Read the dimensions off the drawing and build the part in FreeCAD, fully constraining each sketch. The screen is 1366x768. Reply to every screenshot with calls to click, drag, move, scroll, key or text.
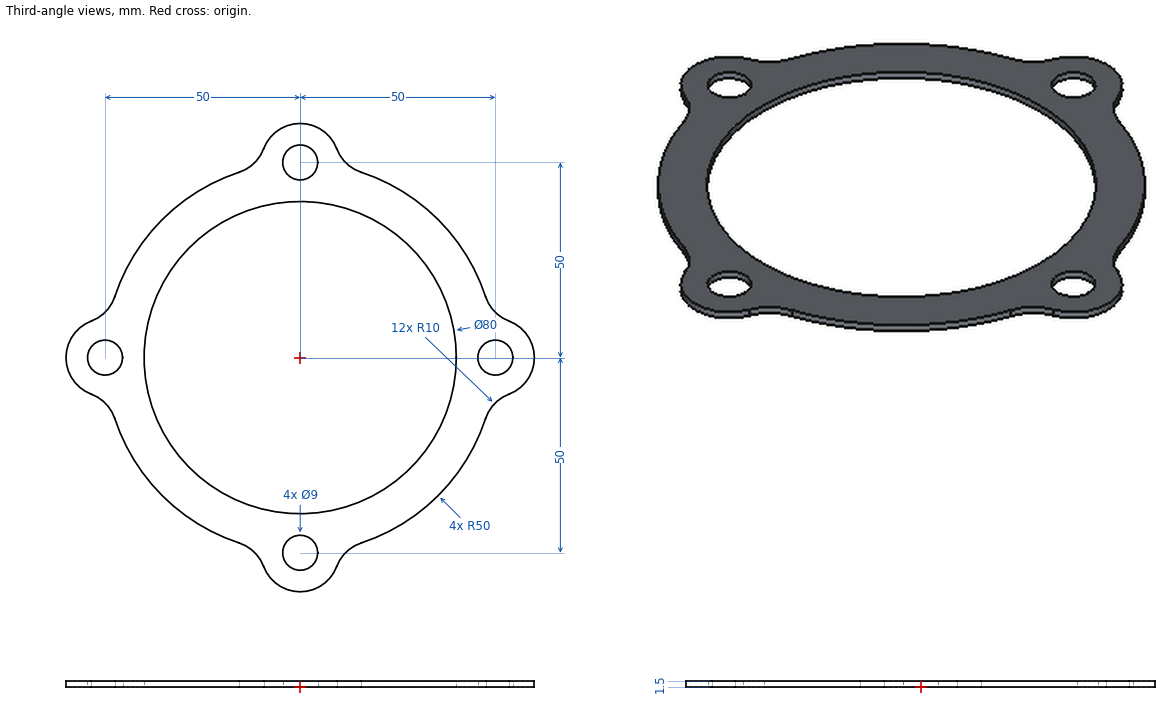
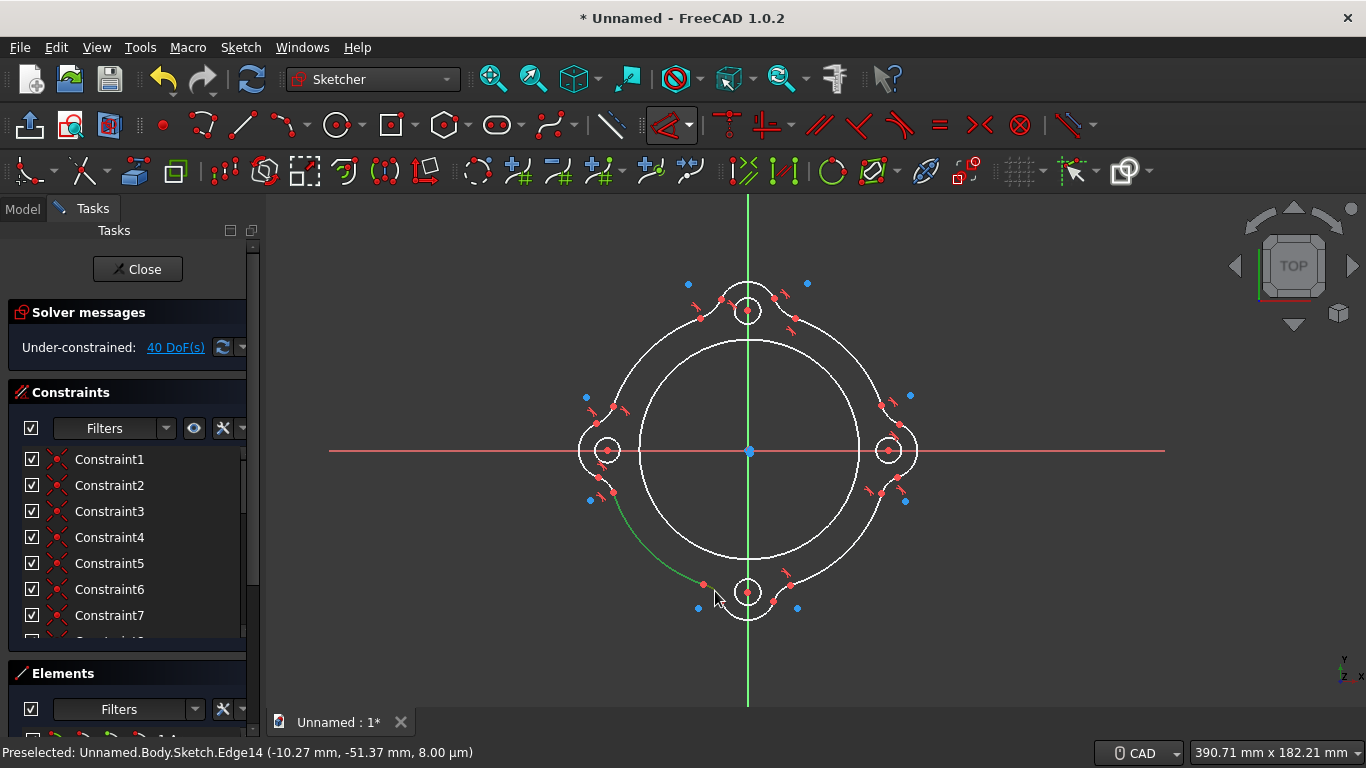
click(900, 126)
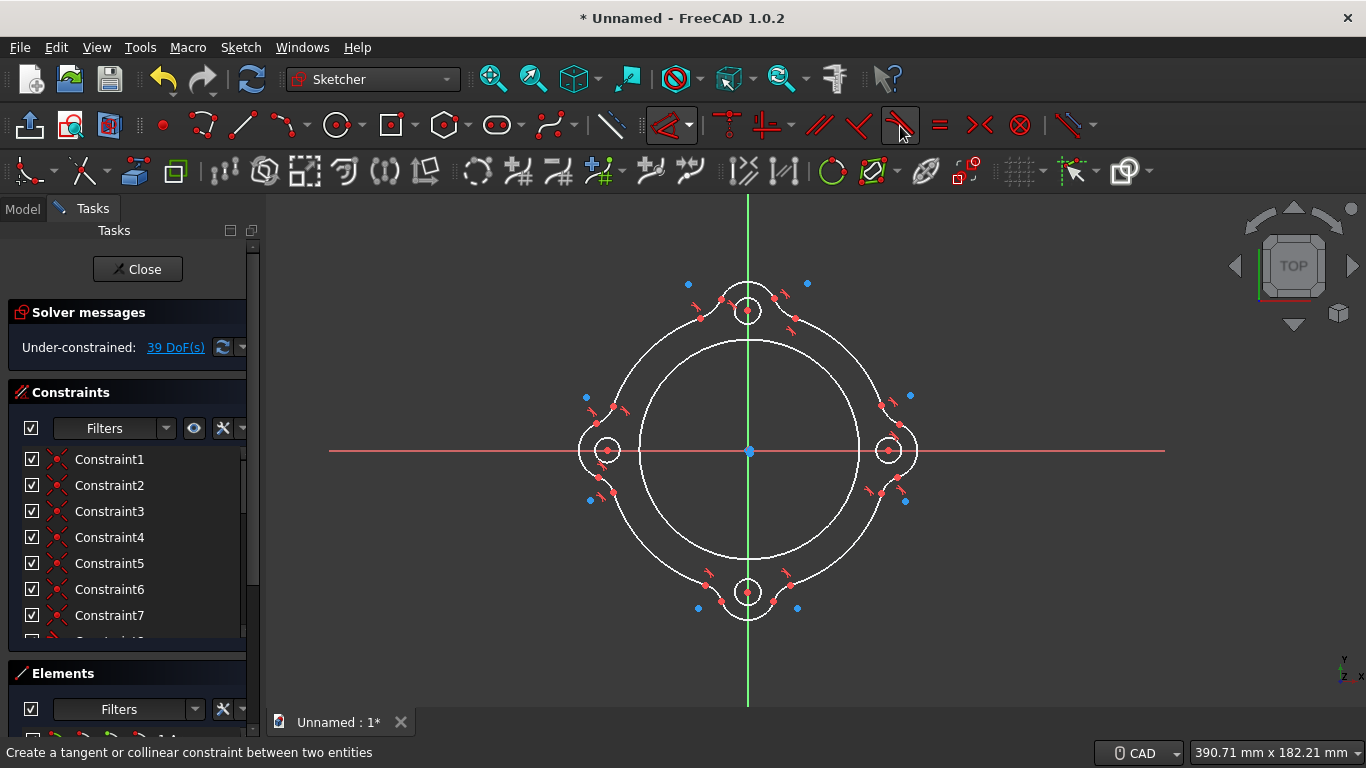
click(716, 591)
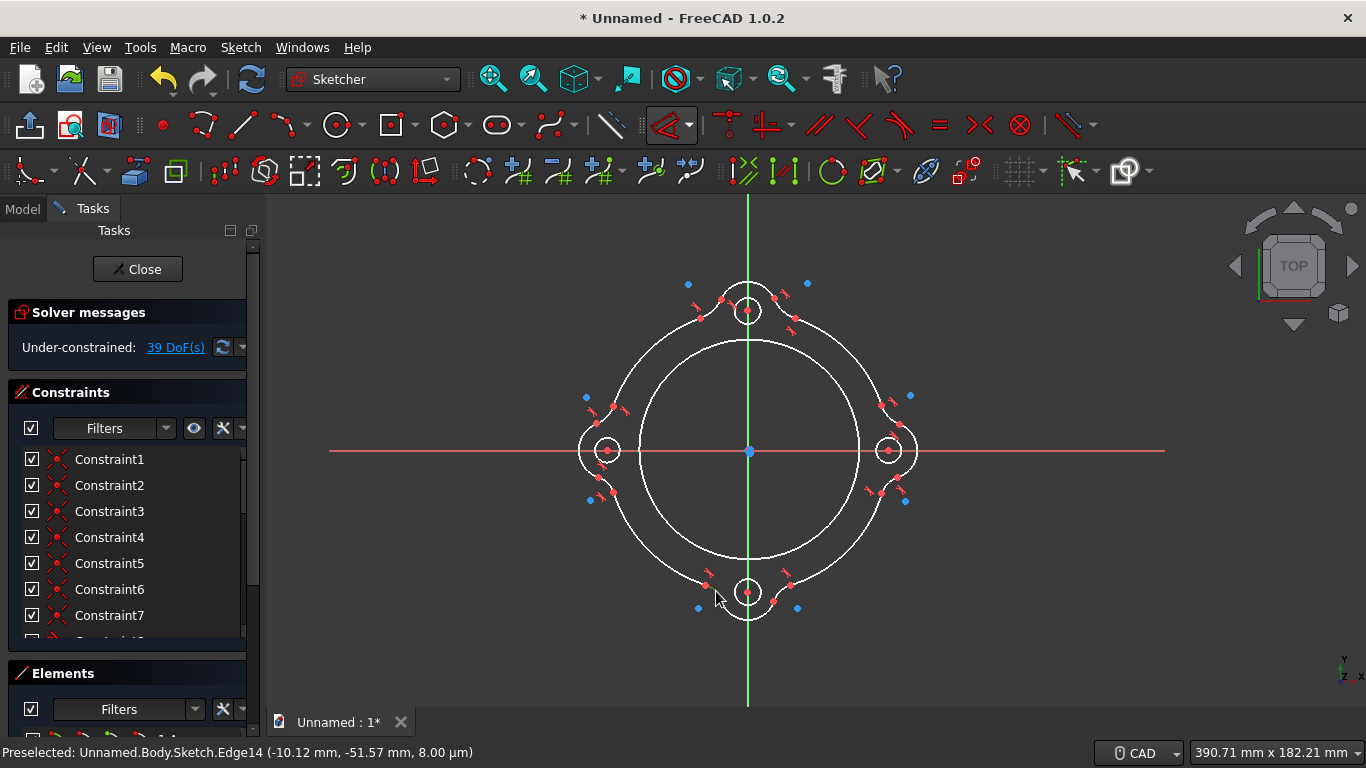
click(735, 617)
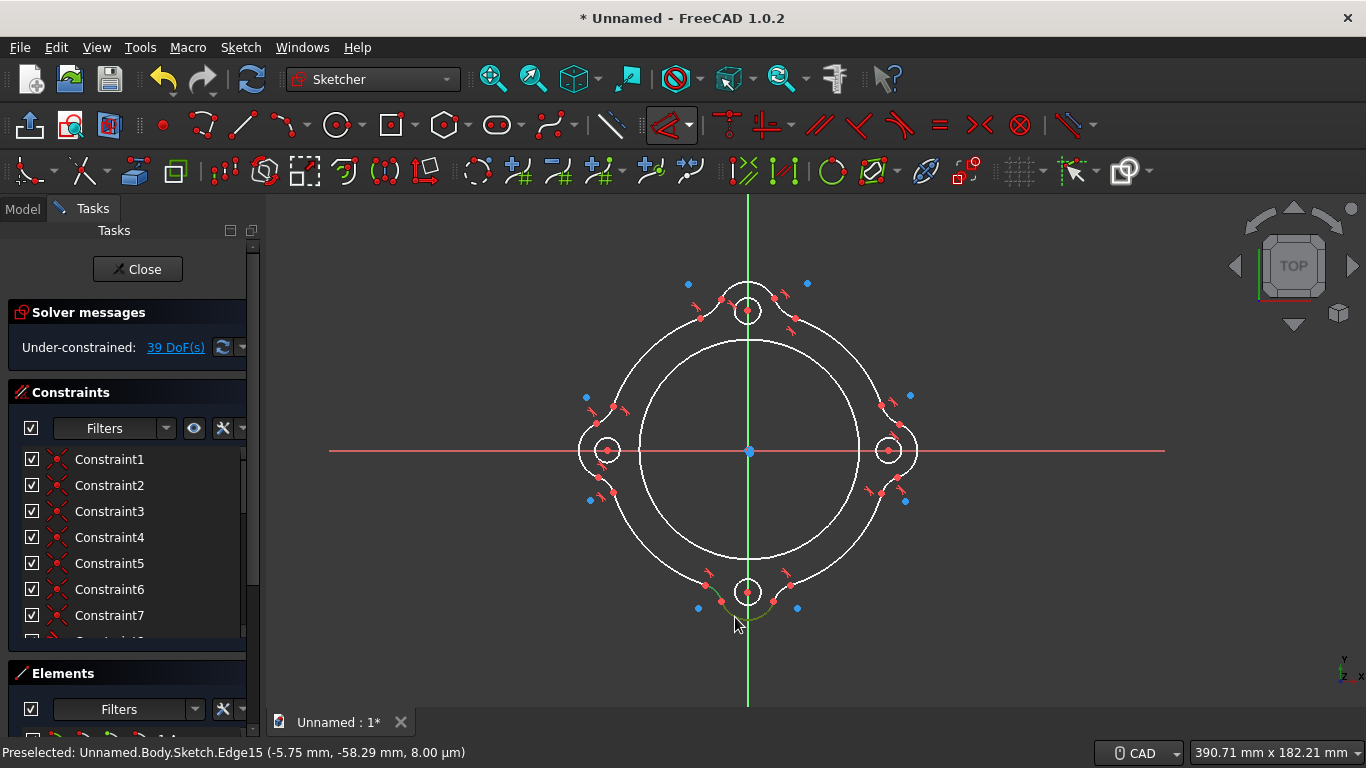
click(900, 126)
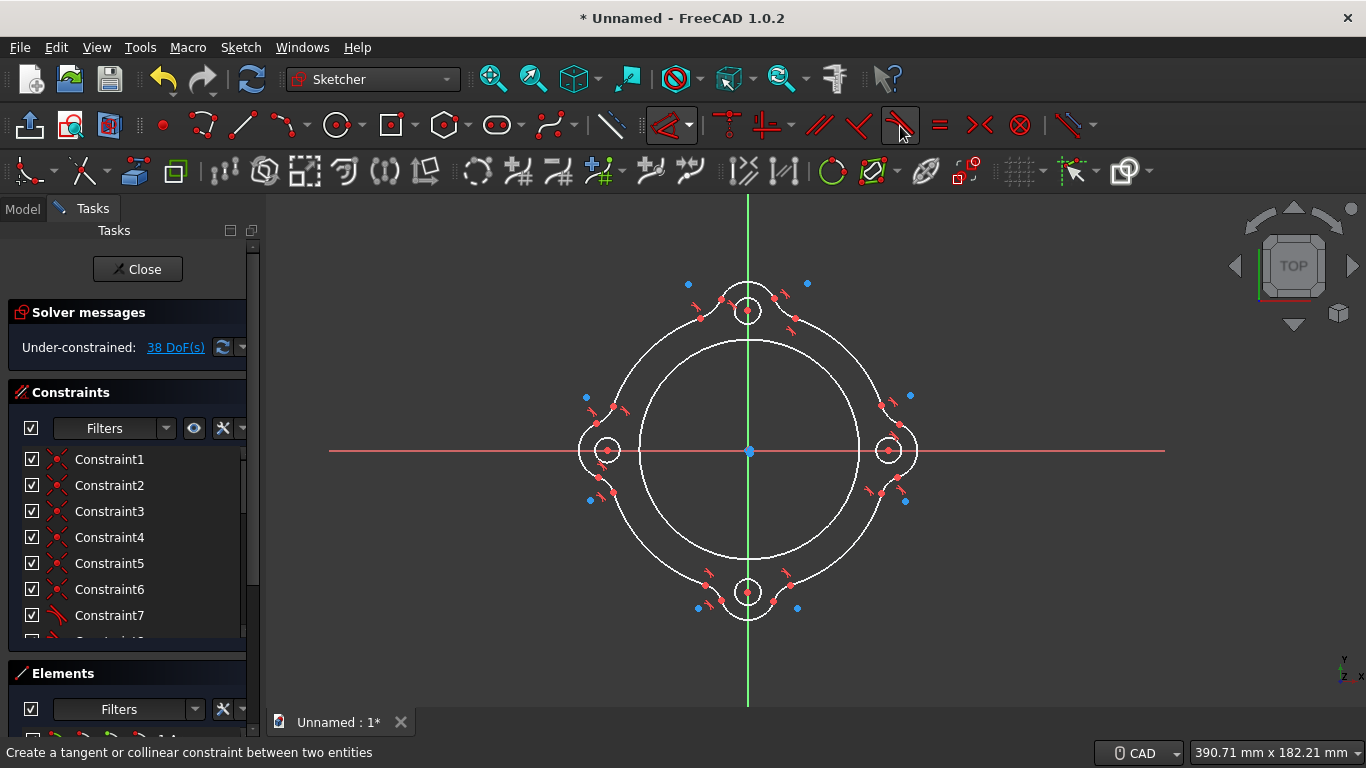
click(734, 616)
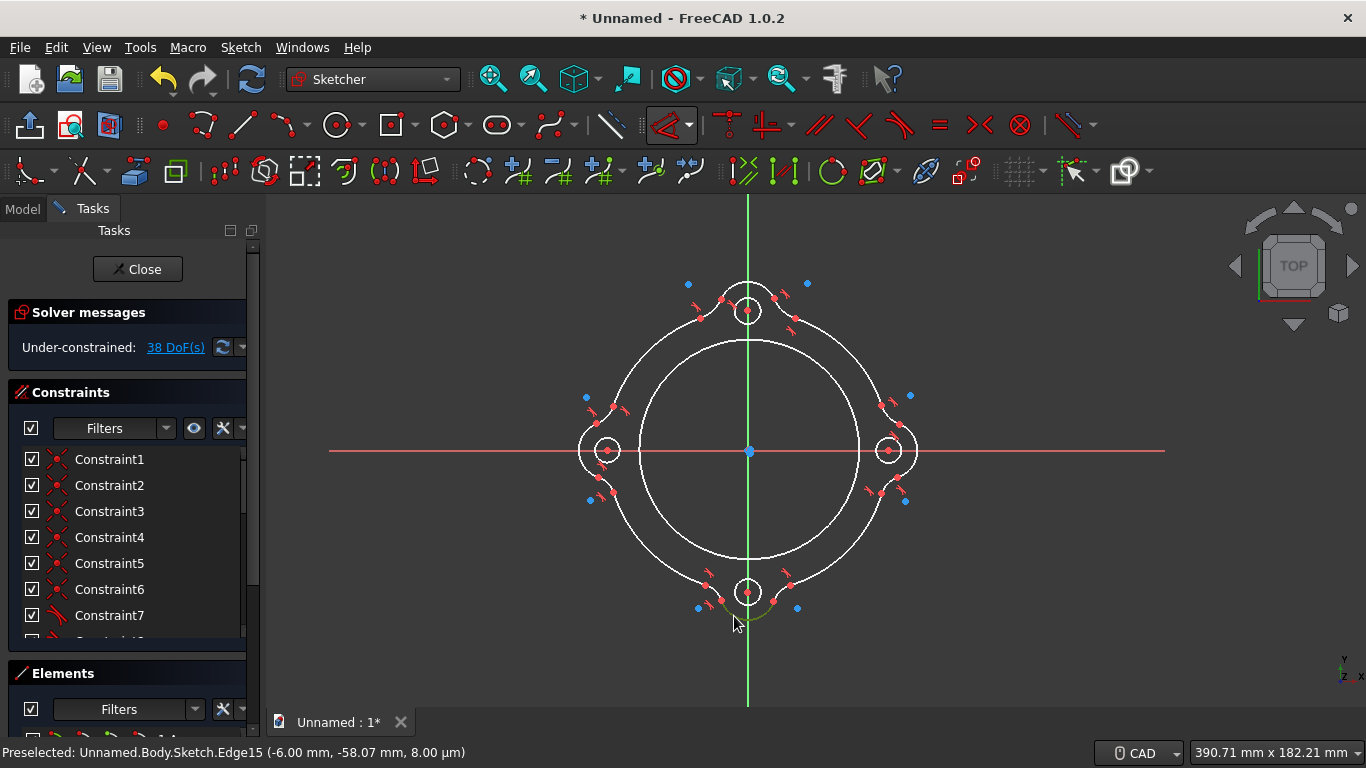
click(780, 592)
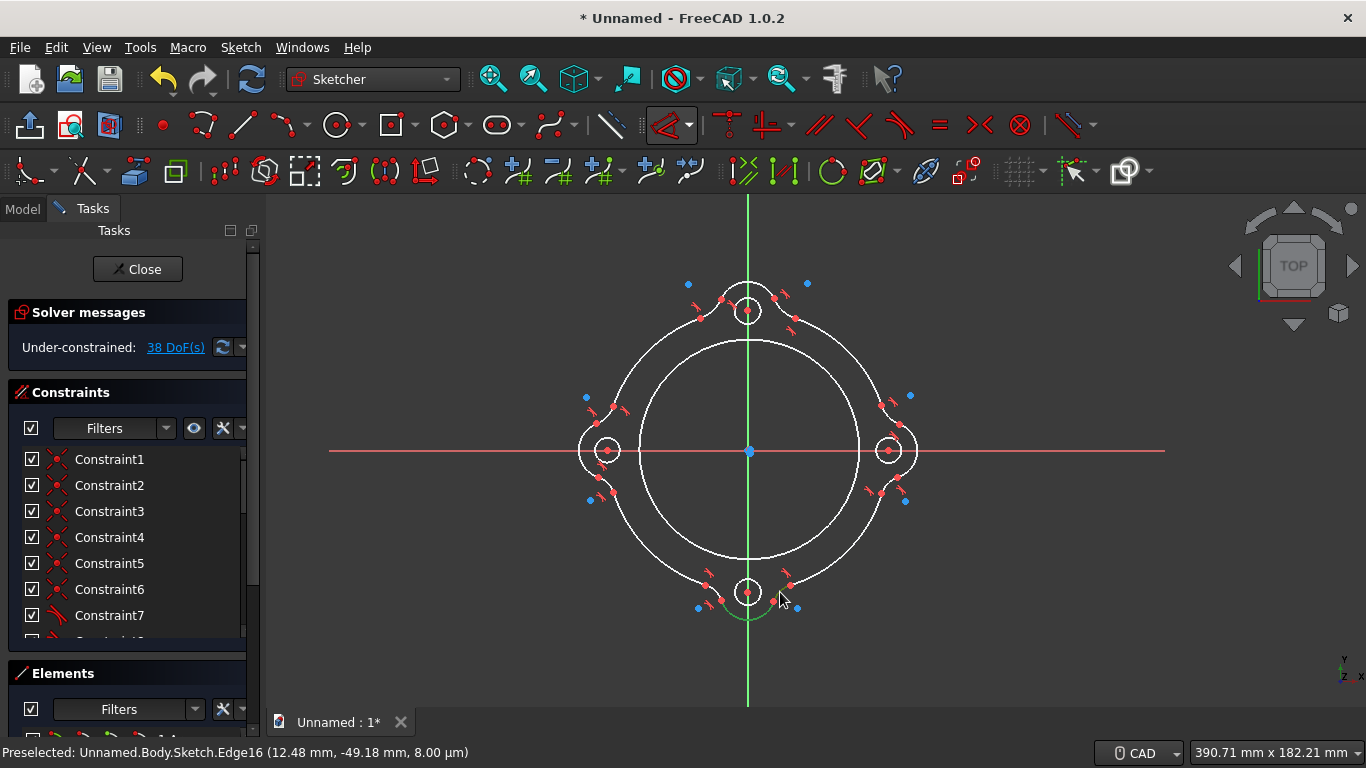
click(900, 126)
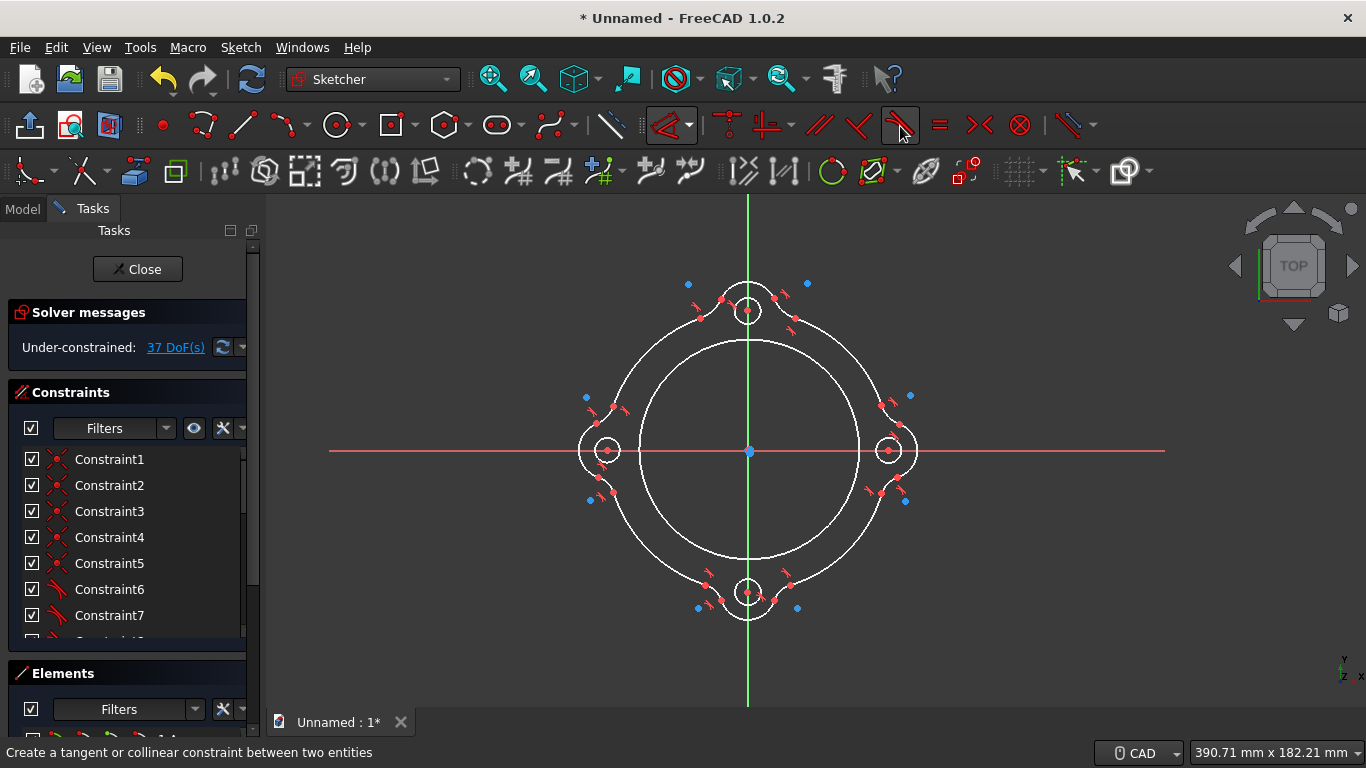
click(827, 371)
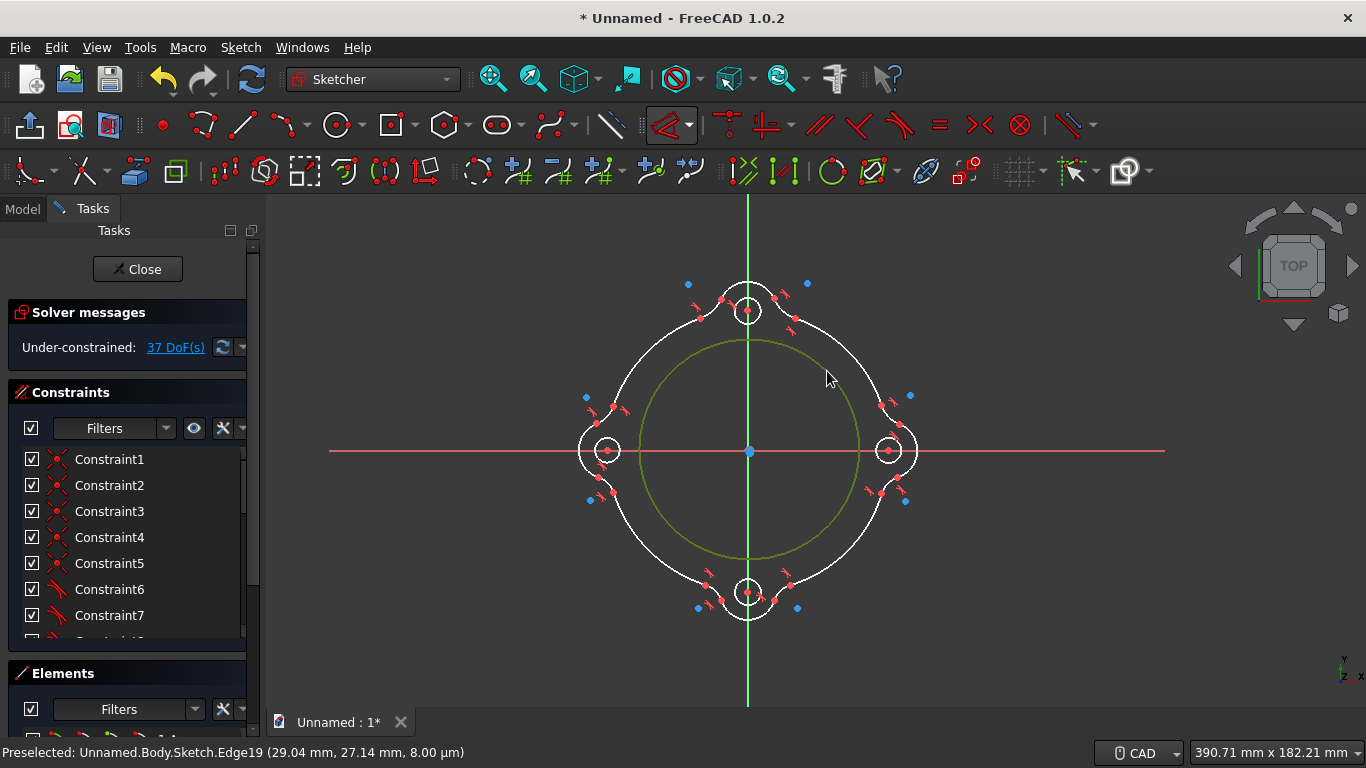
click(827, 568)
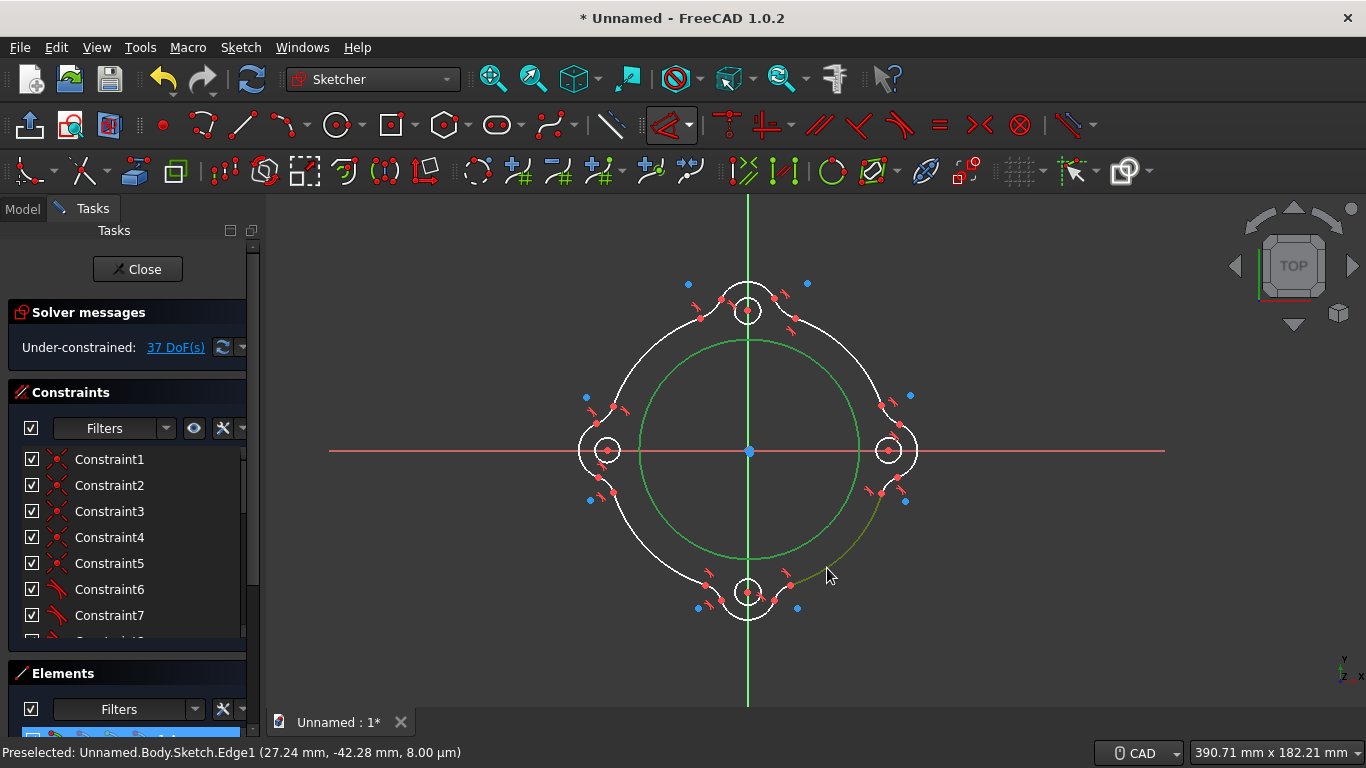
click(728, 126)